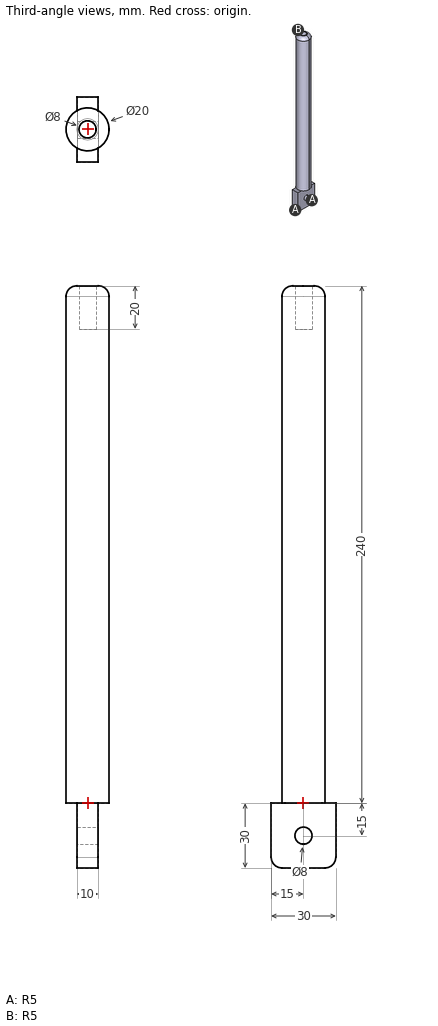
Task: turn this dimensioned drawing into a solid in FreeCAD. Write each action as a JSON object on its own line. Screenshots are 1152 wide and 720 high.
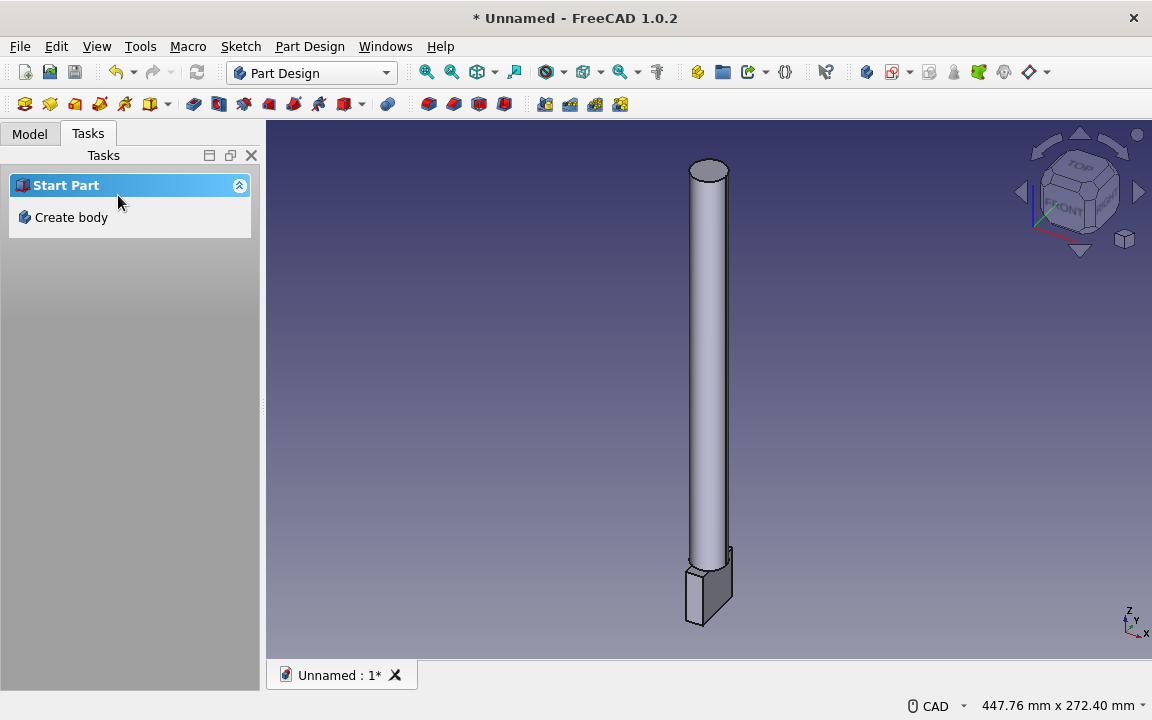
{"action": "left_click", "coordinate": [718, 586]}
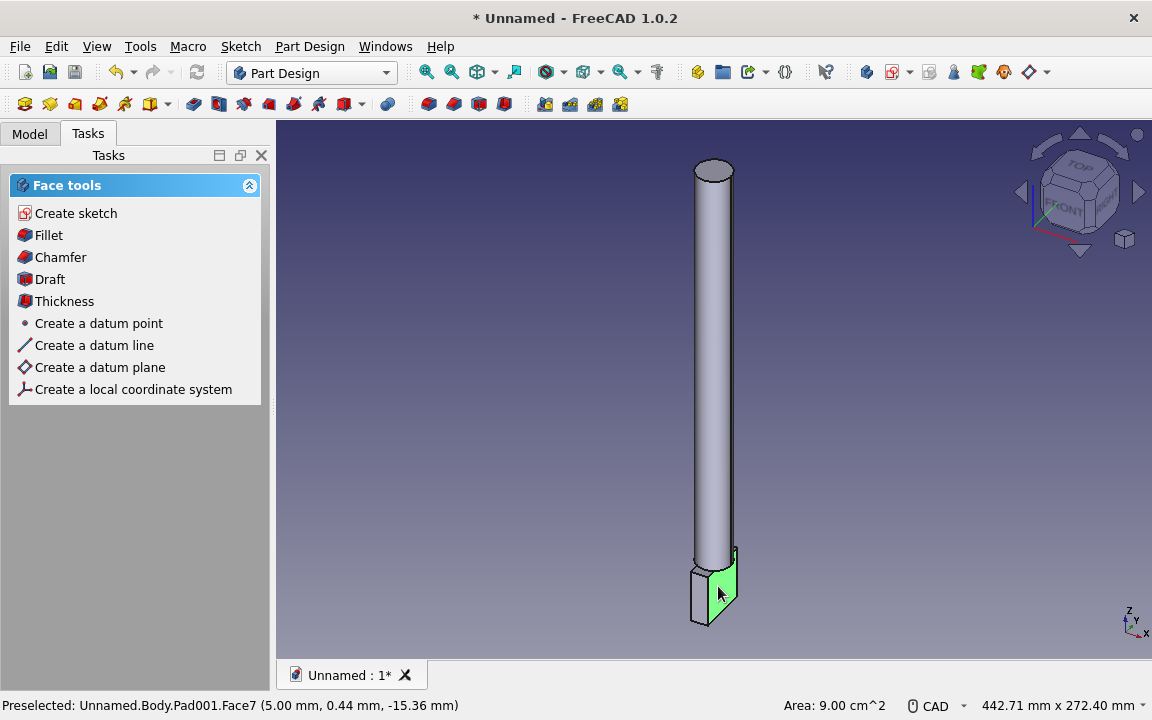
{"action": "left_click", "coordinate": [892, 72]}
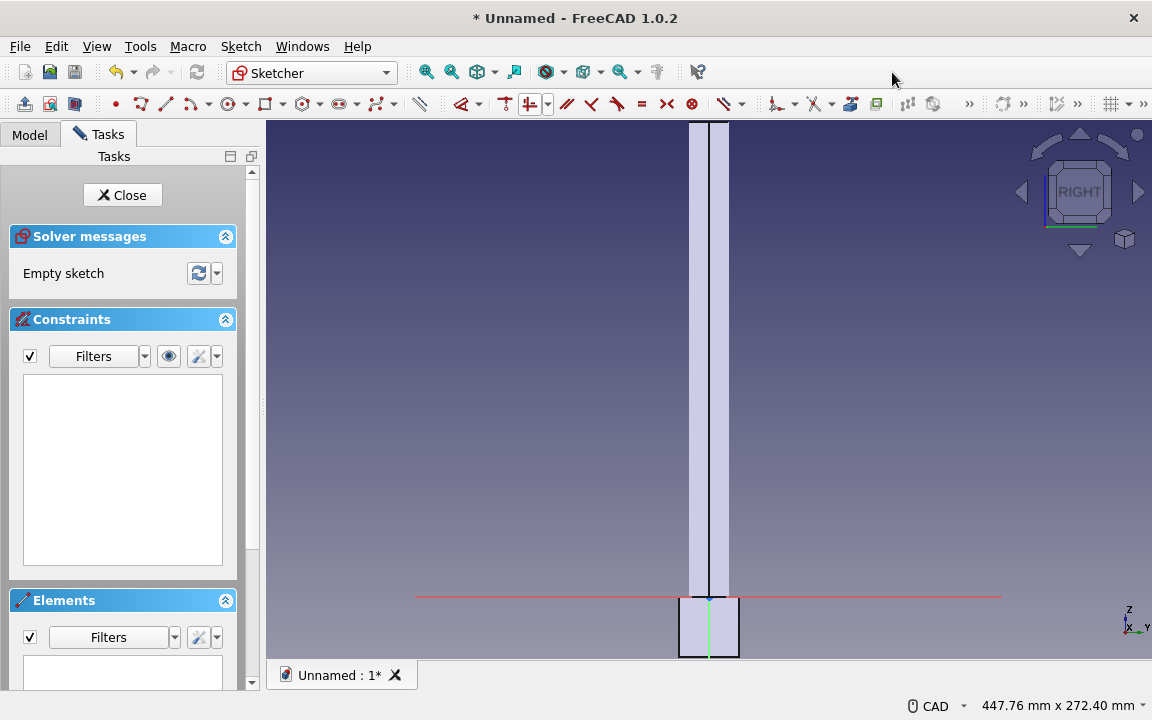
{"action": "key", "text": "q s"}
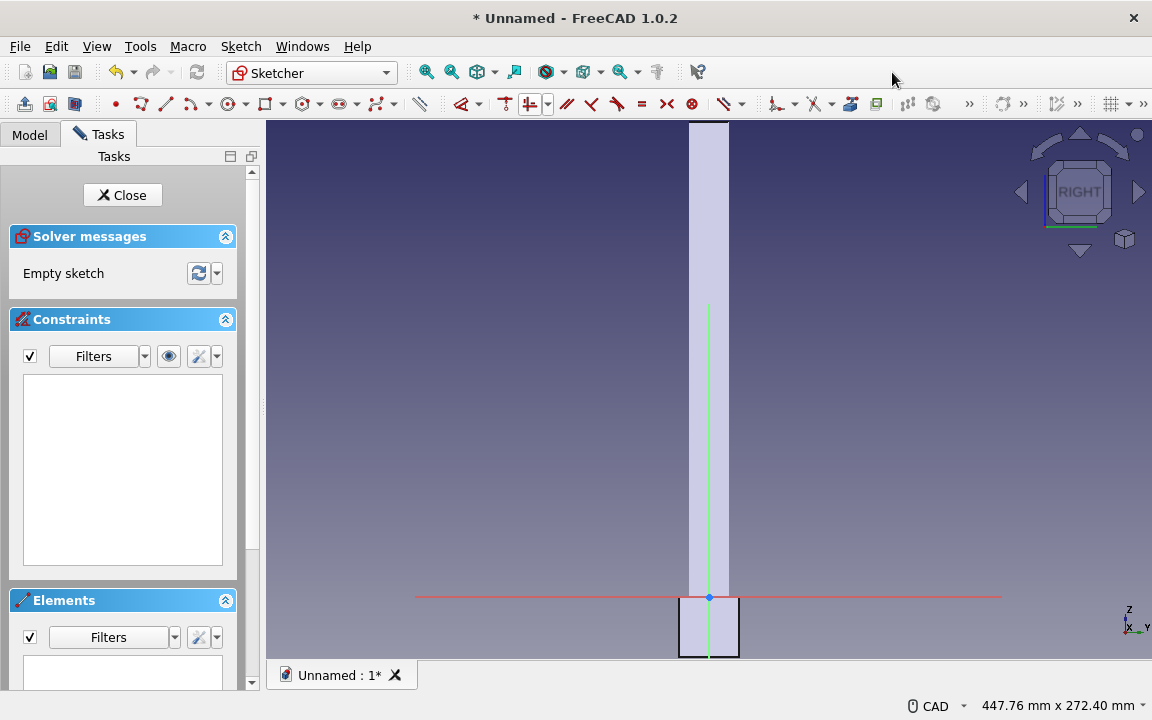
{"action": "scroll", "coordinate": [640, 390], "scroll_direction": "down", "scroll_amount": 5}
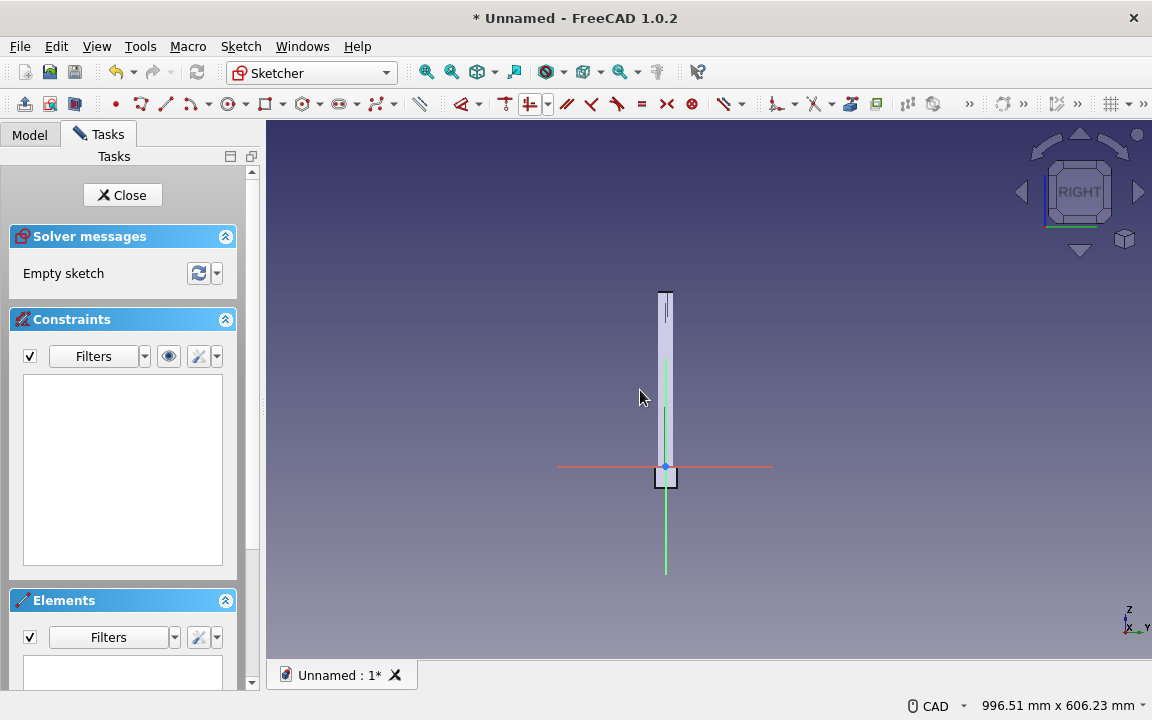
{"action": "scroll", "coordinate": [667, 478], "scroll_direction": "up", "scroll_amount": 15}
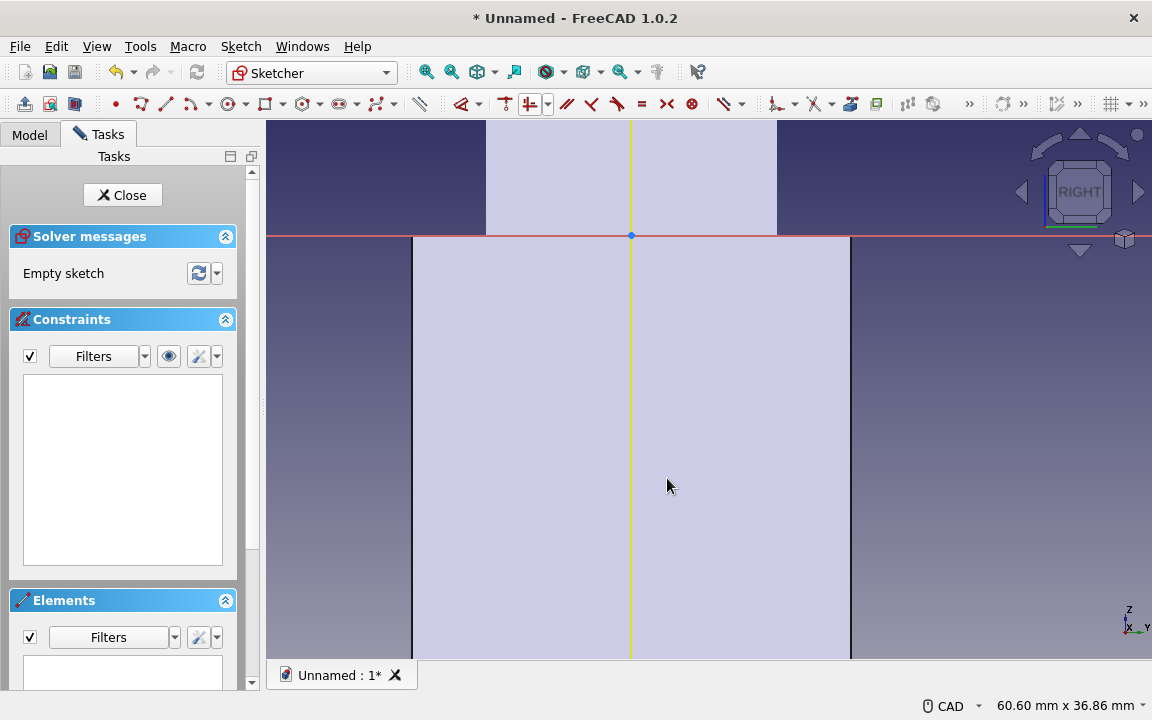
{"action": "key", "text": "g c"}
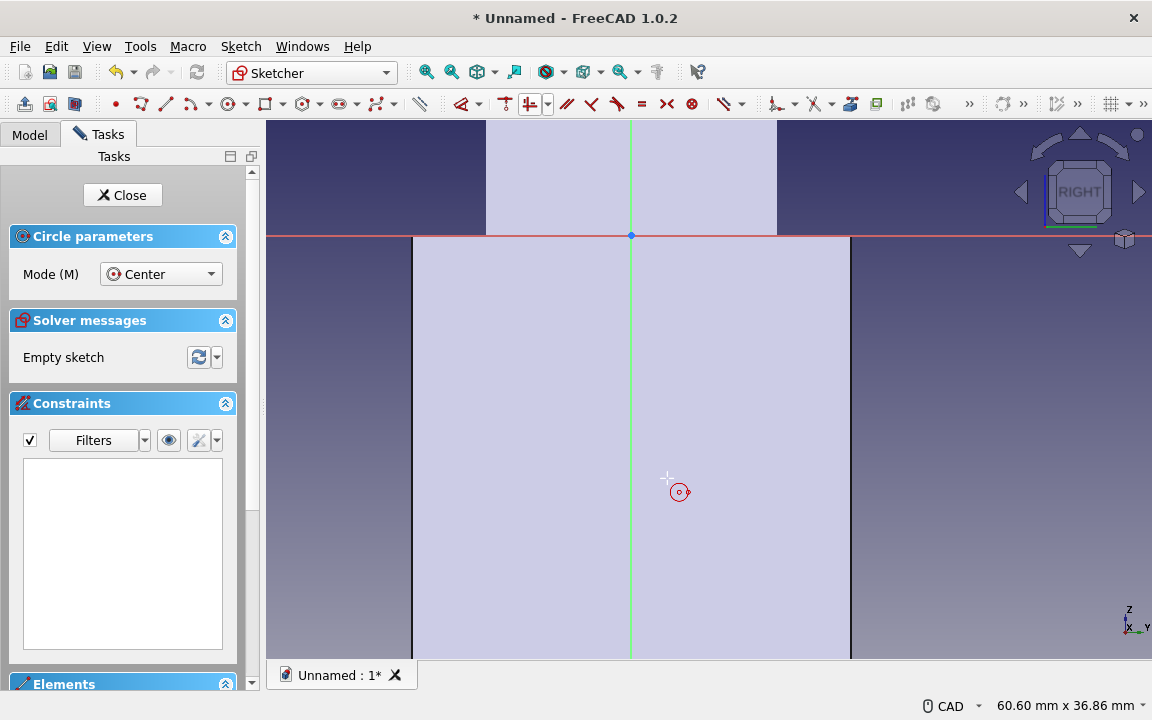
{"action": "left_click", "coordinate": [631, 455]}
{"action": "left_click", "coordinate": [673, 414]}
{"action": "key", "text": "Escape"}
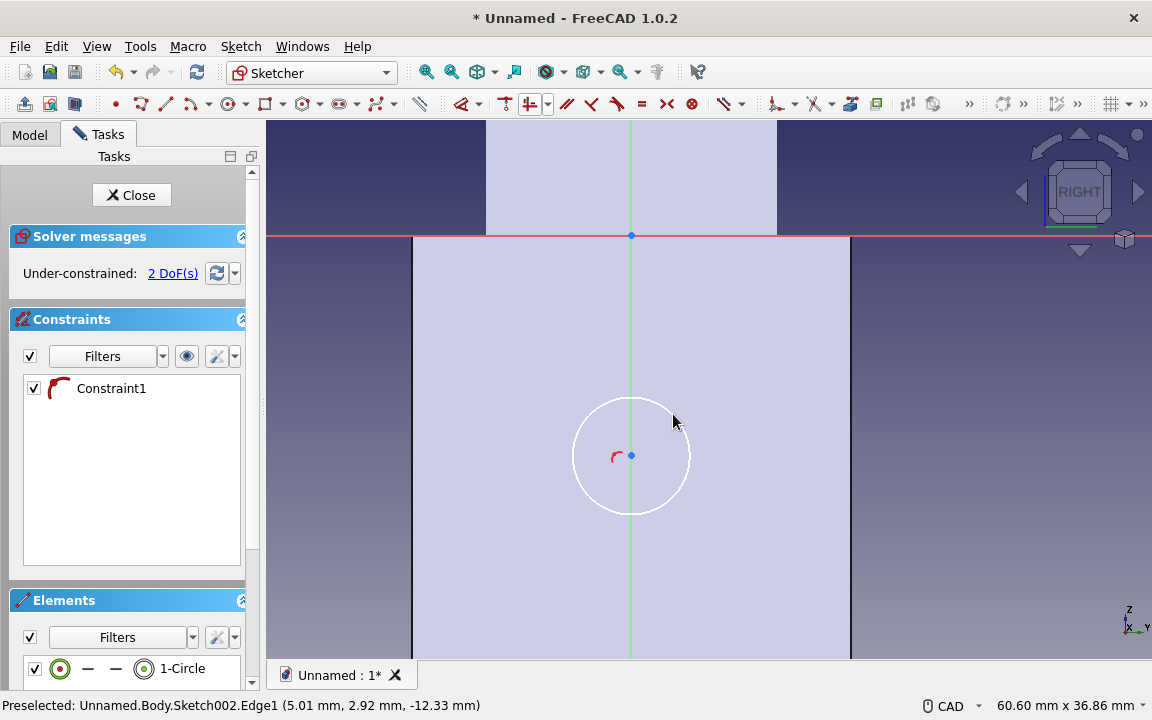
{"action": "key", "text": "d"}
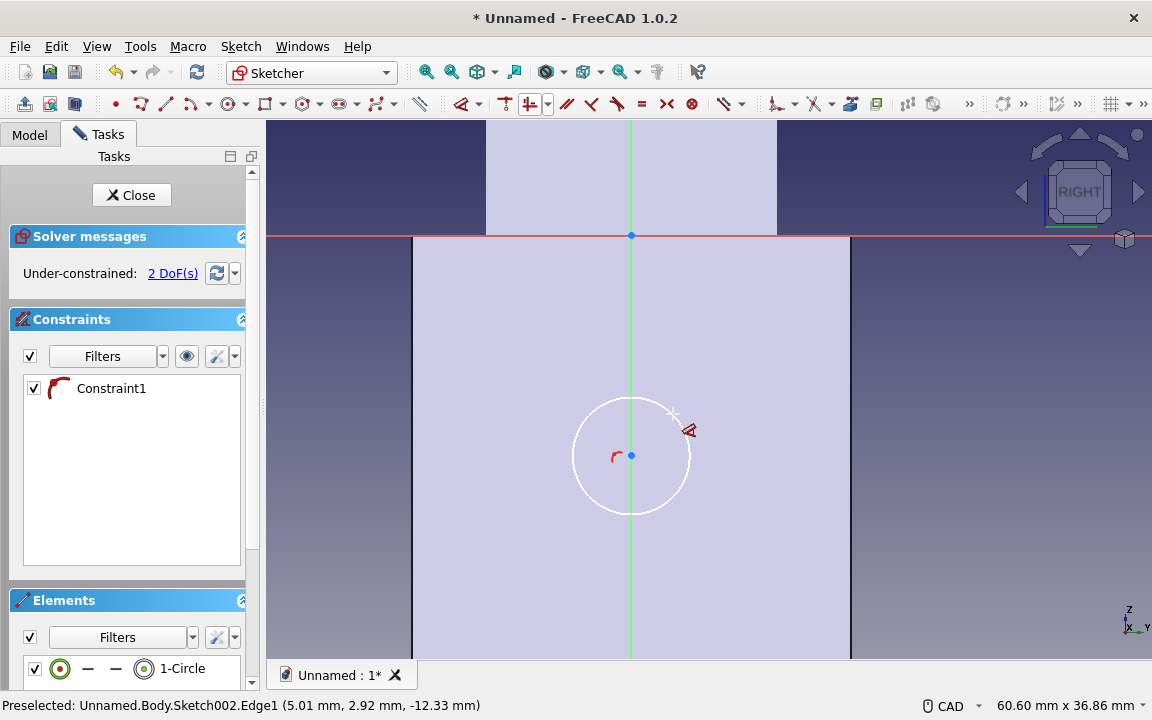
{"action": "left_click", "coordinate": [672, 414]}
{"action": "left_click", "coordinate": [694, 391]}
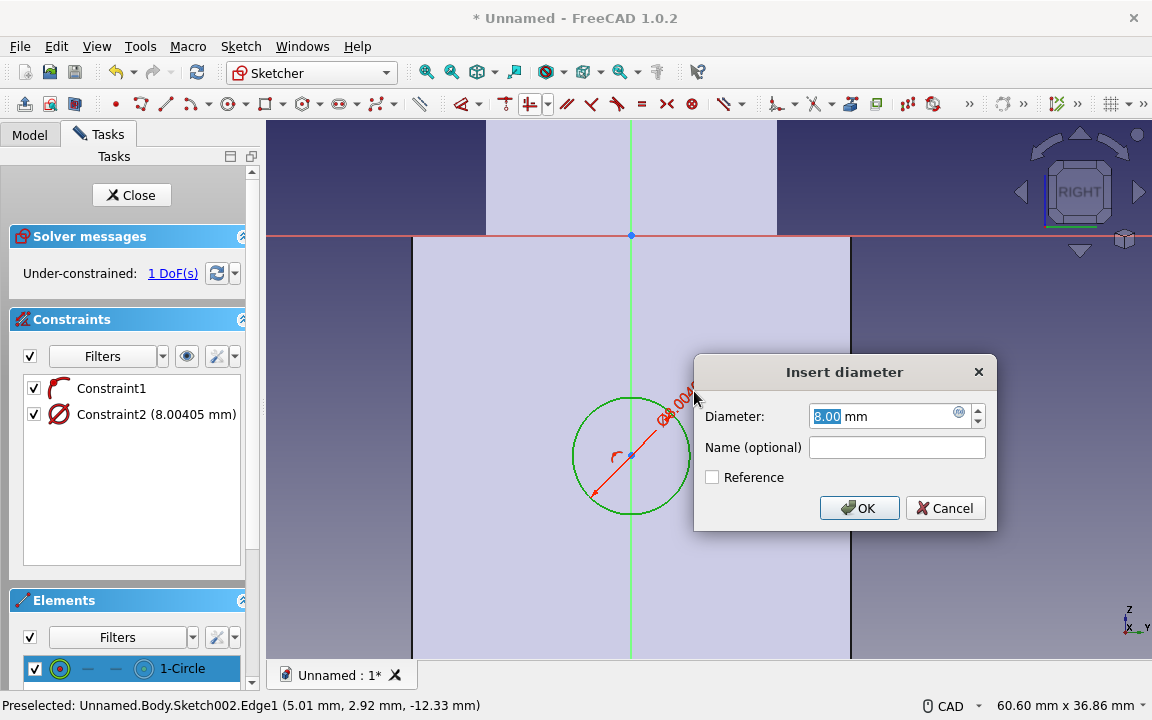
{"action": "type", "text": "8"}
{"action": "key", "text": "Return"}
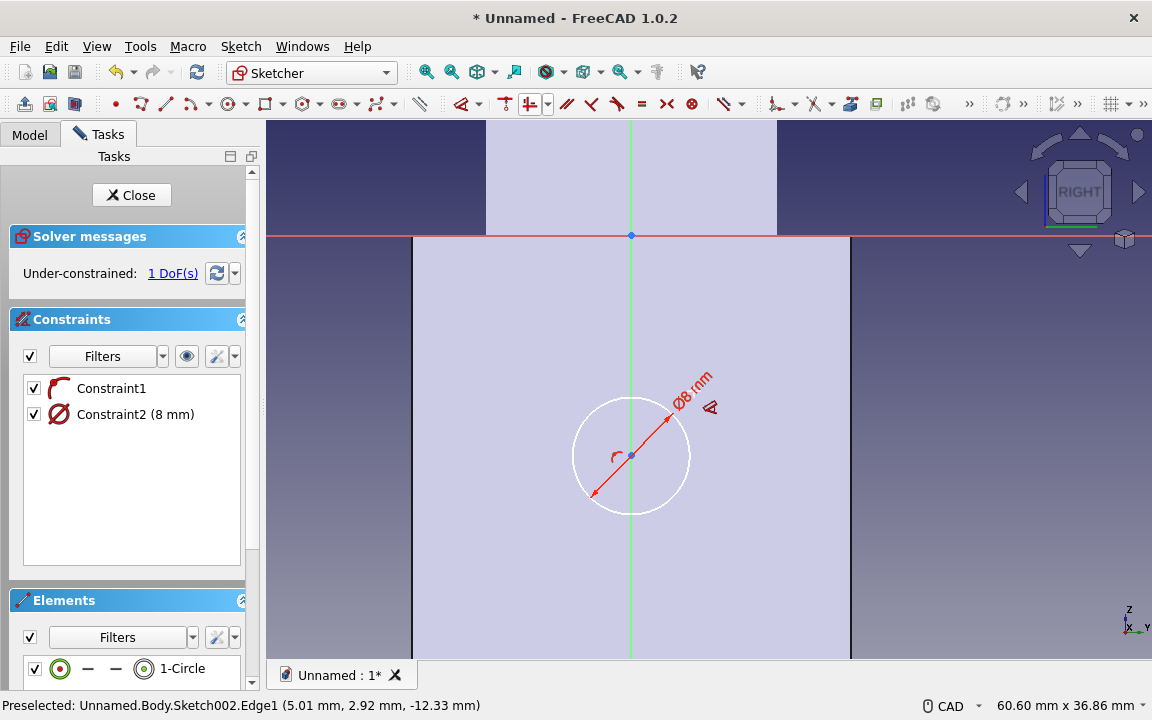
{"action": "left_click", "coordinate": [631, 456]}
{"action": "left_click", "coordinate": [665, 346]}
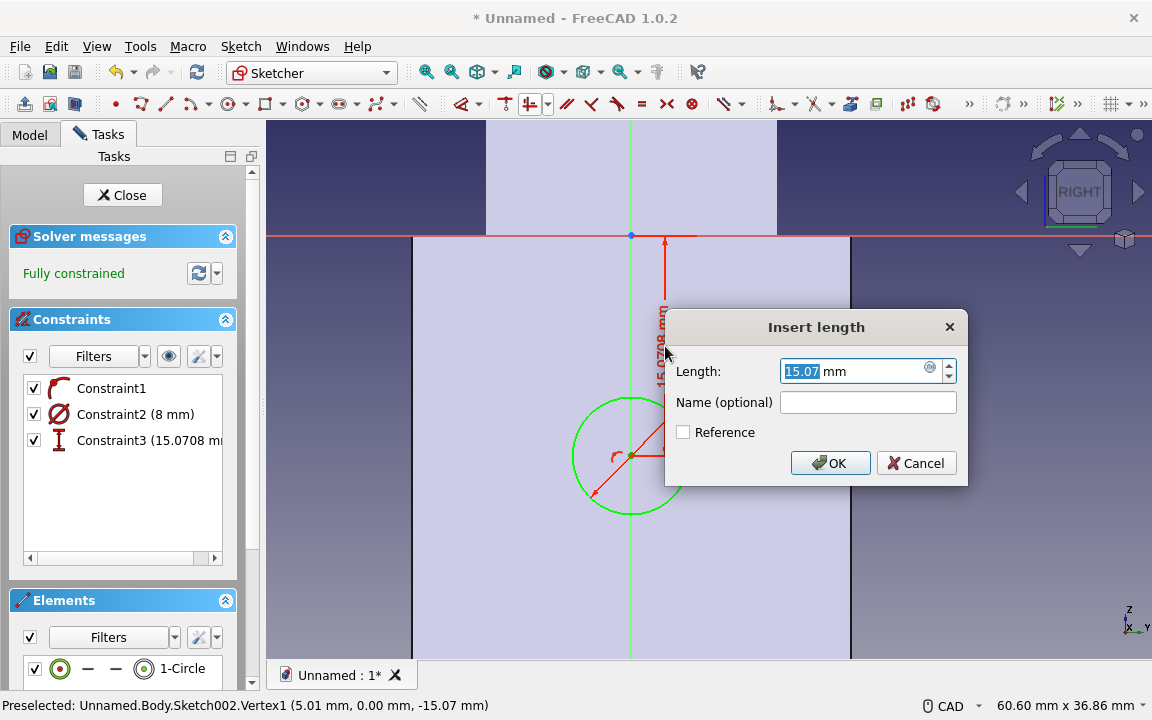
{"action": "type", "text": "15"}
{"action": "key", "text": "Return"}
{"action": "key", "text": "Escape"}